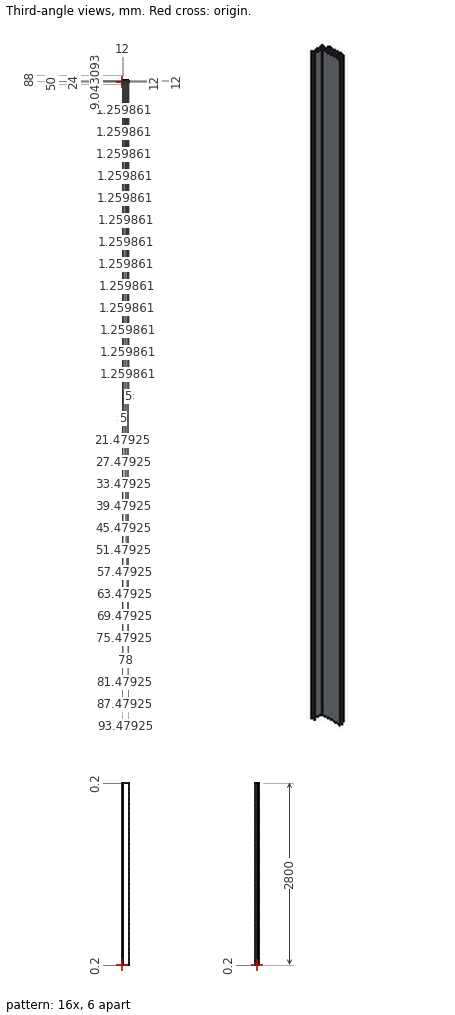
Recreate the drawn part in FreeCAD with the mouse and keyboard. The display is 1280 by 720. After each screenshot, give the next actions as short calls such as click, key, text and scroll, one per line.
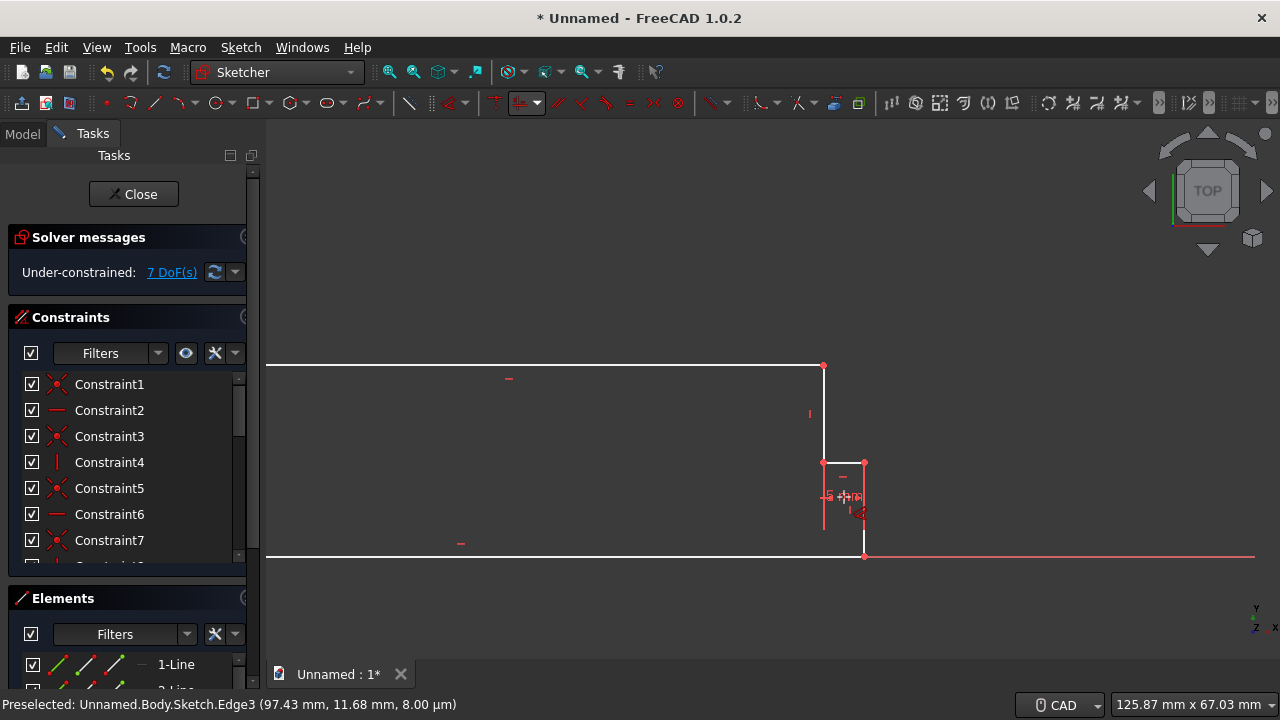
scroll(902, 581, down, 4)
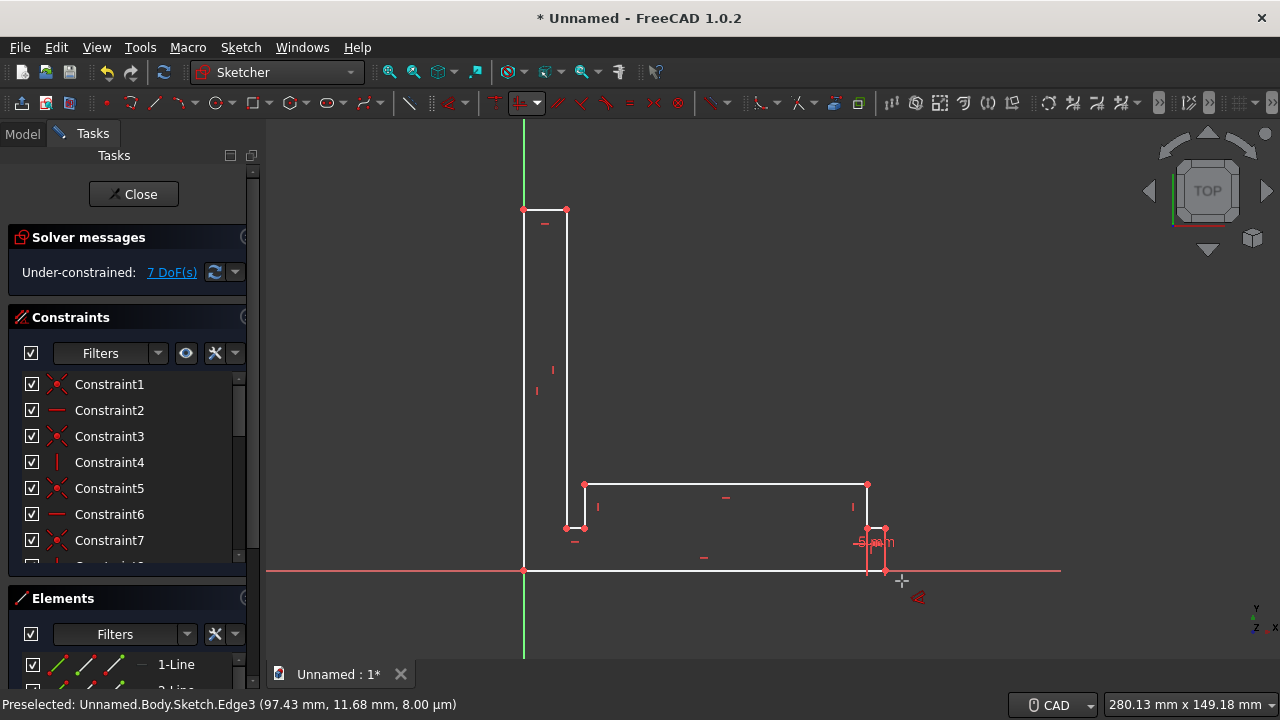
scroll(579, 528, up, 5)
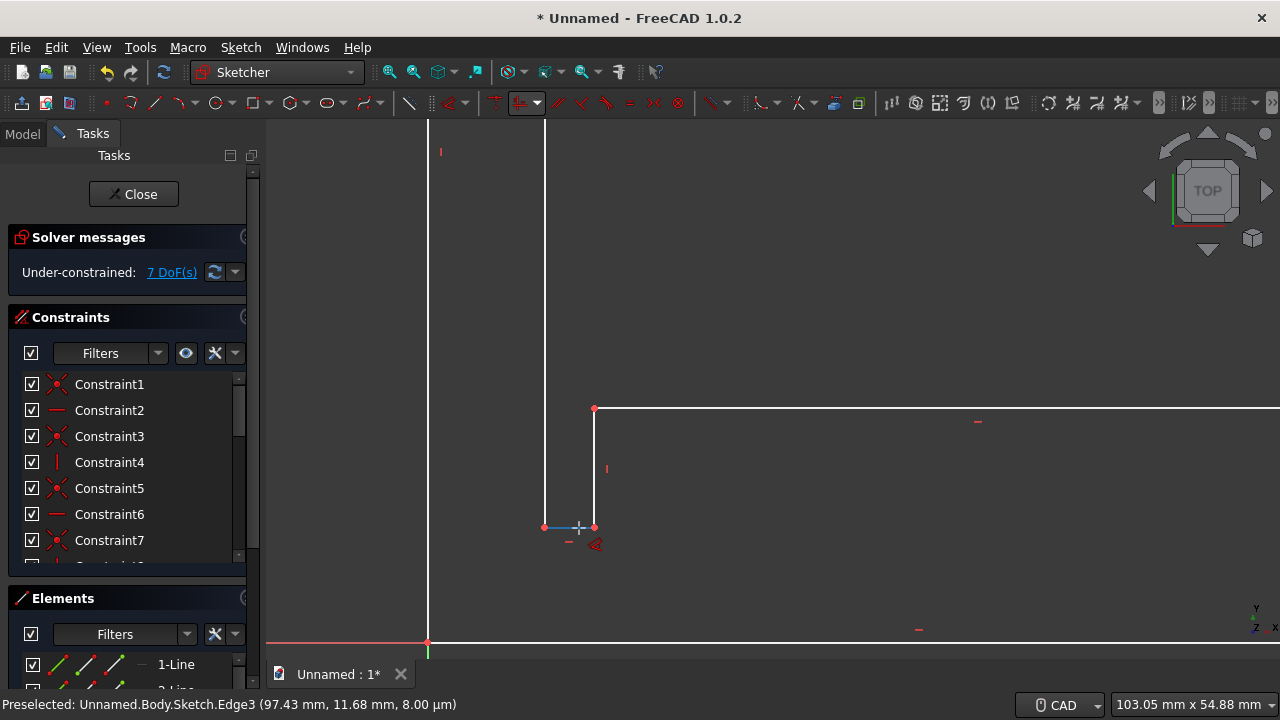
click(579, 528)
click(569, 562)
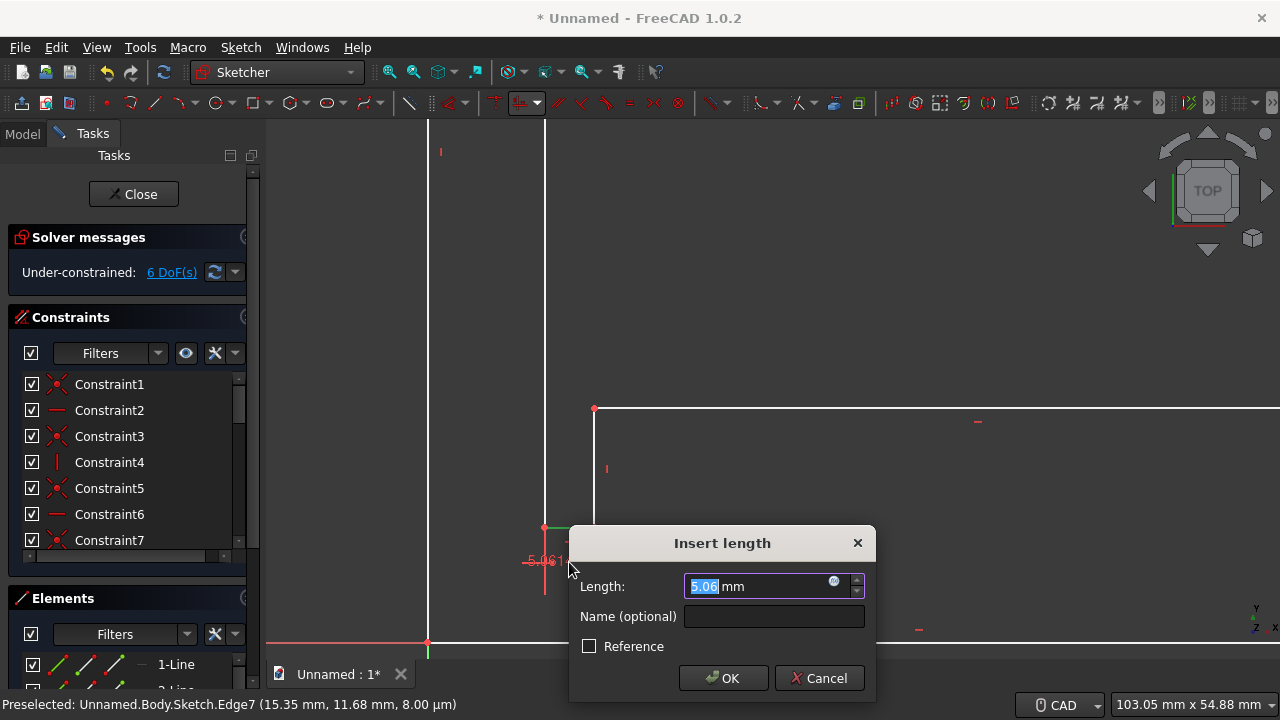
text(5)
key(Return)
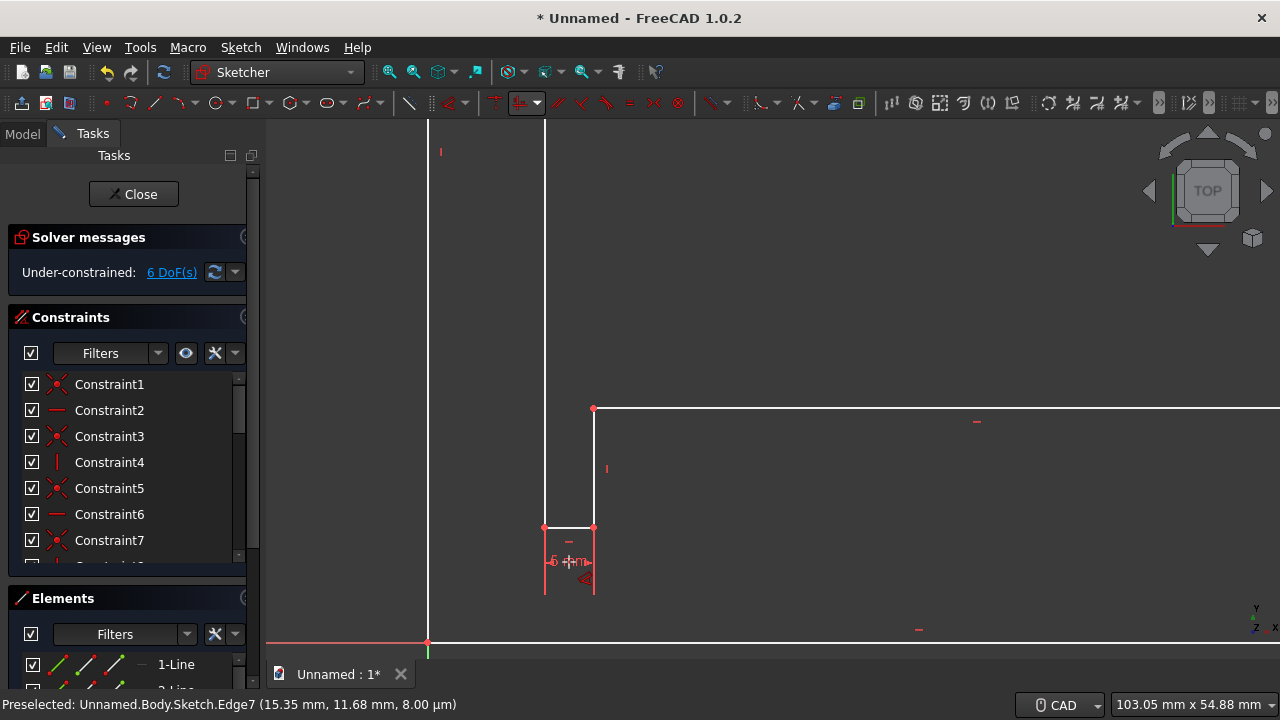
scroll(579, 528, down, 5)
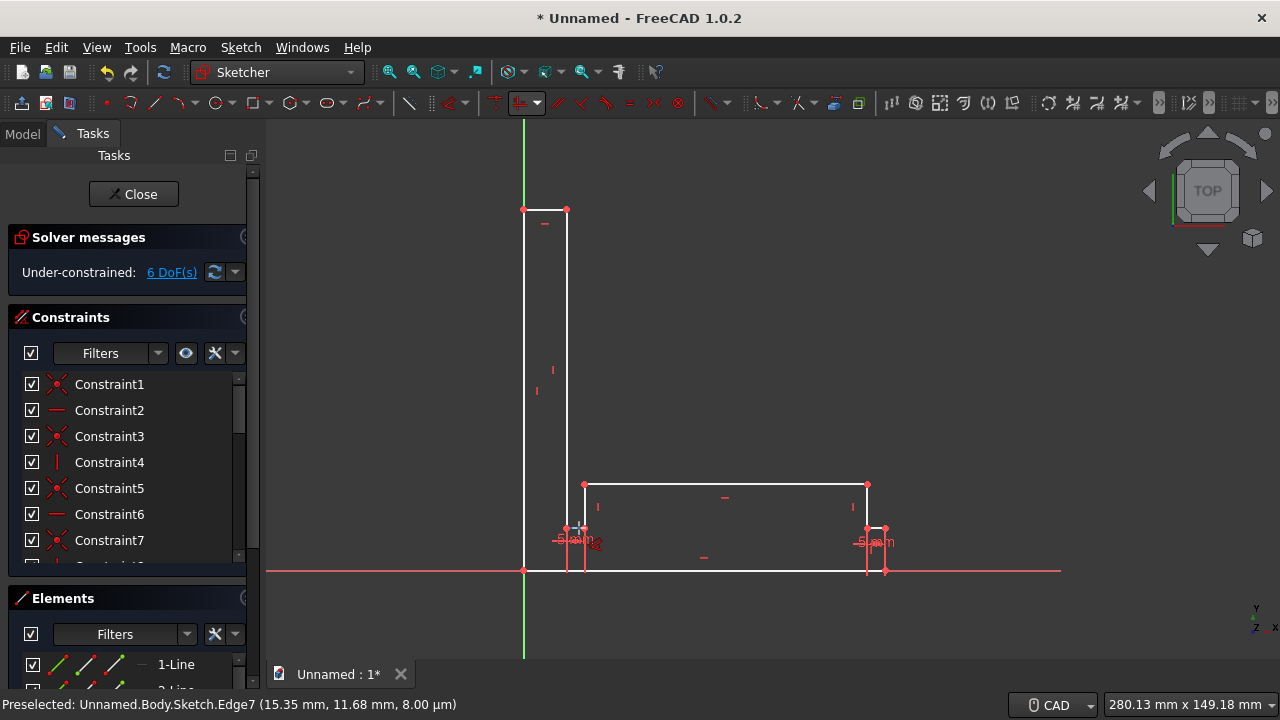
click(885, 558)
click(967, 550)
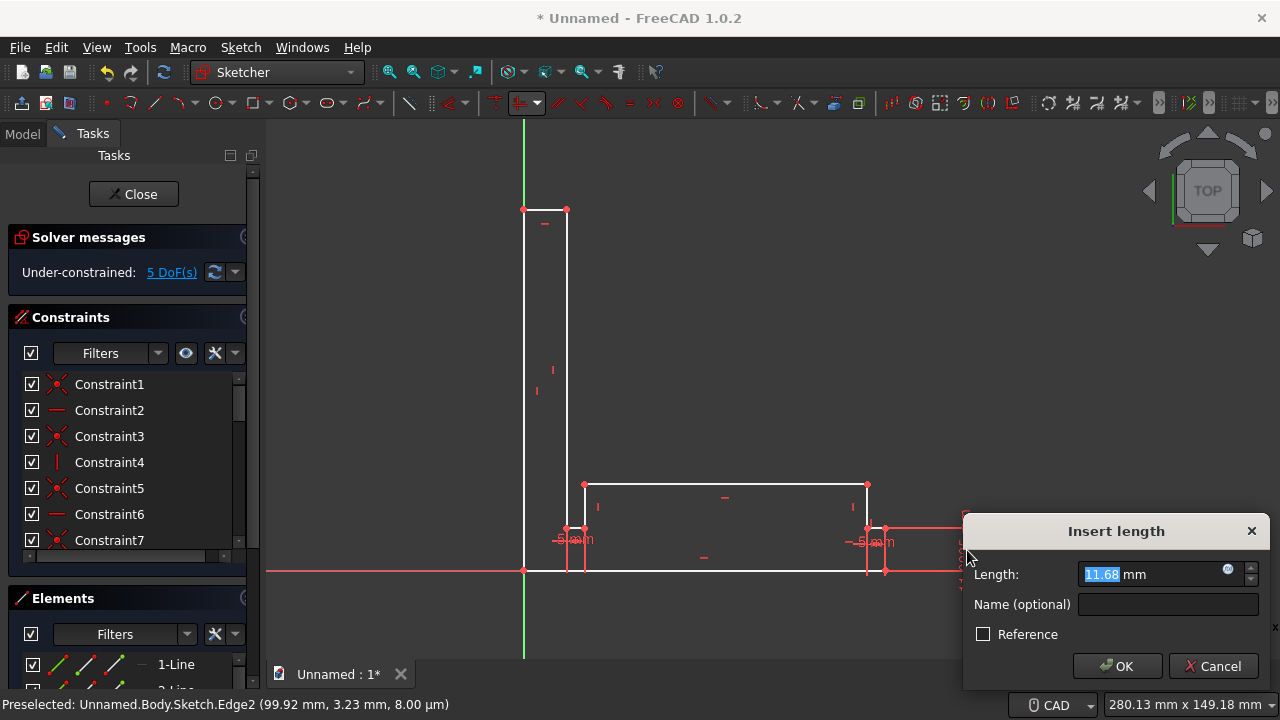
text(12)
key(Return)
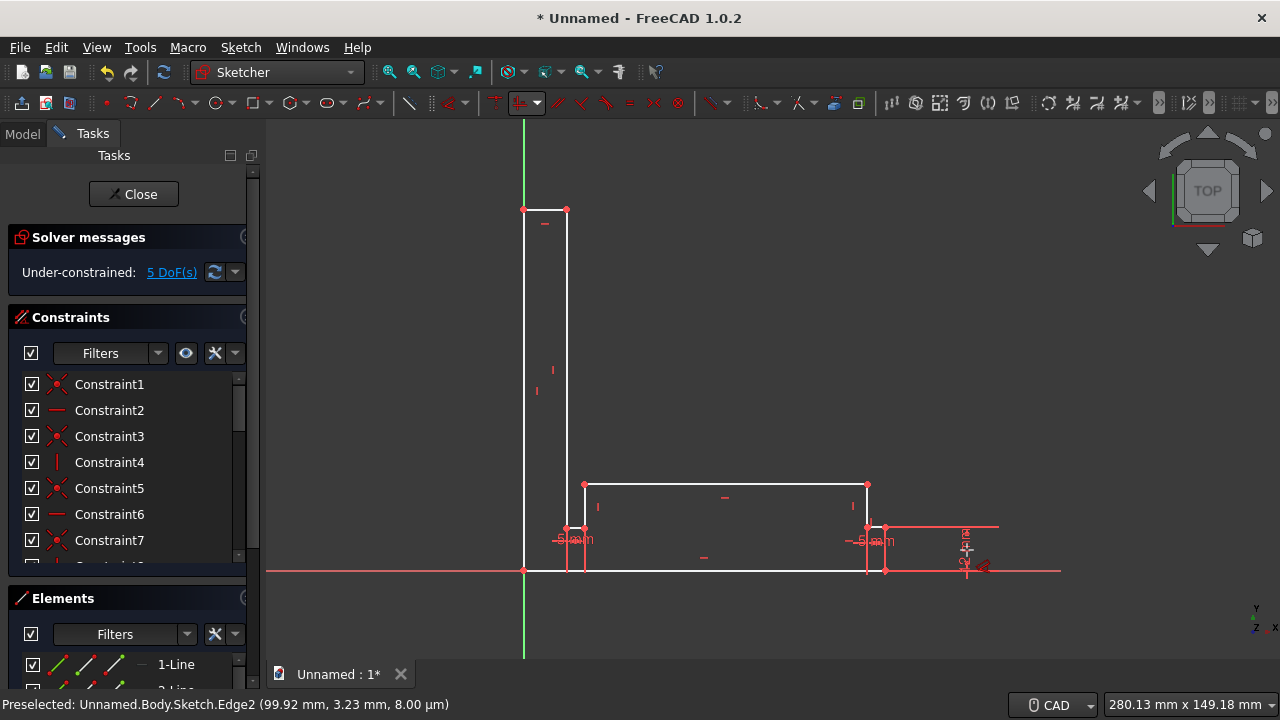
click(867, 514)
click(901, 506)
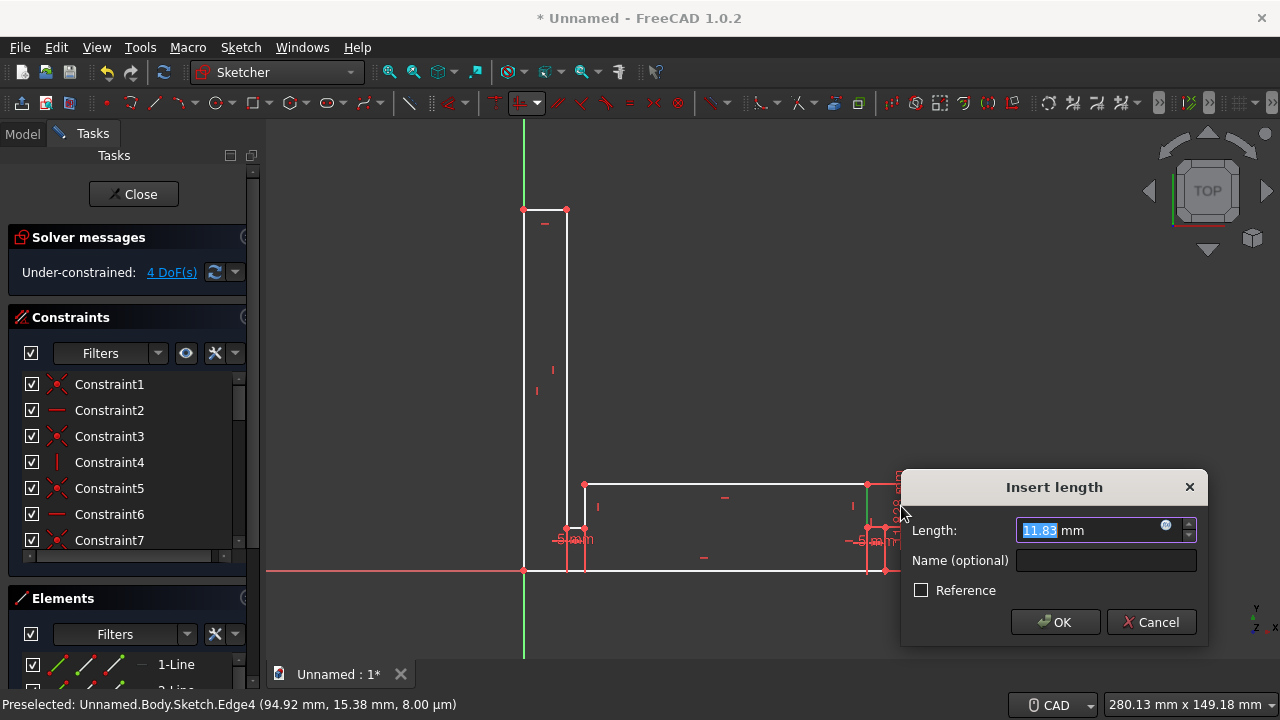
text(12)
key(Return)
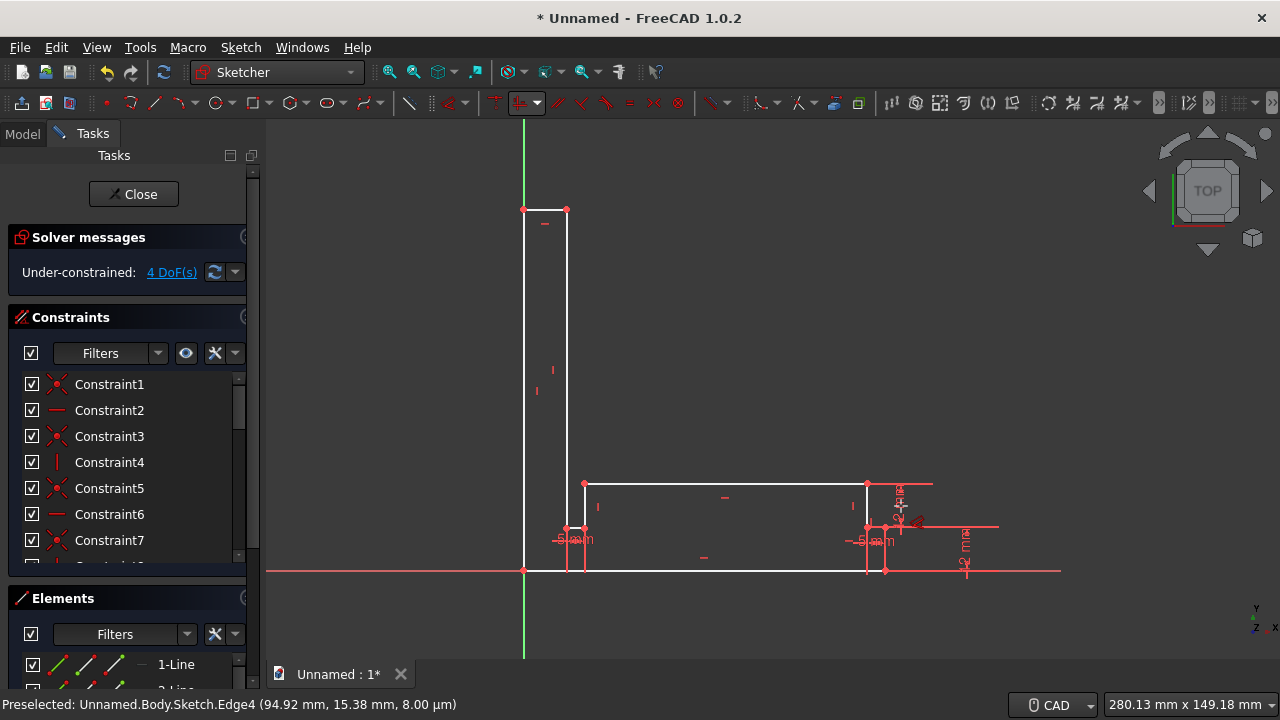
click(782, 484)
click(726, 518)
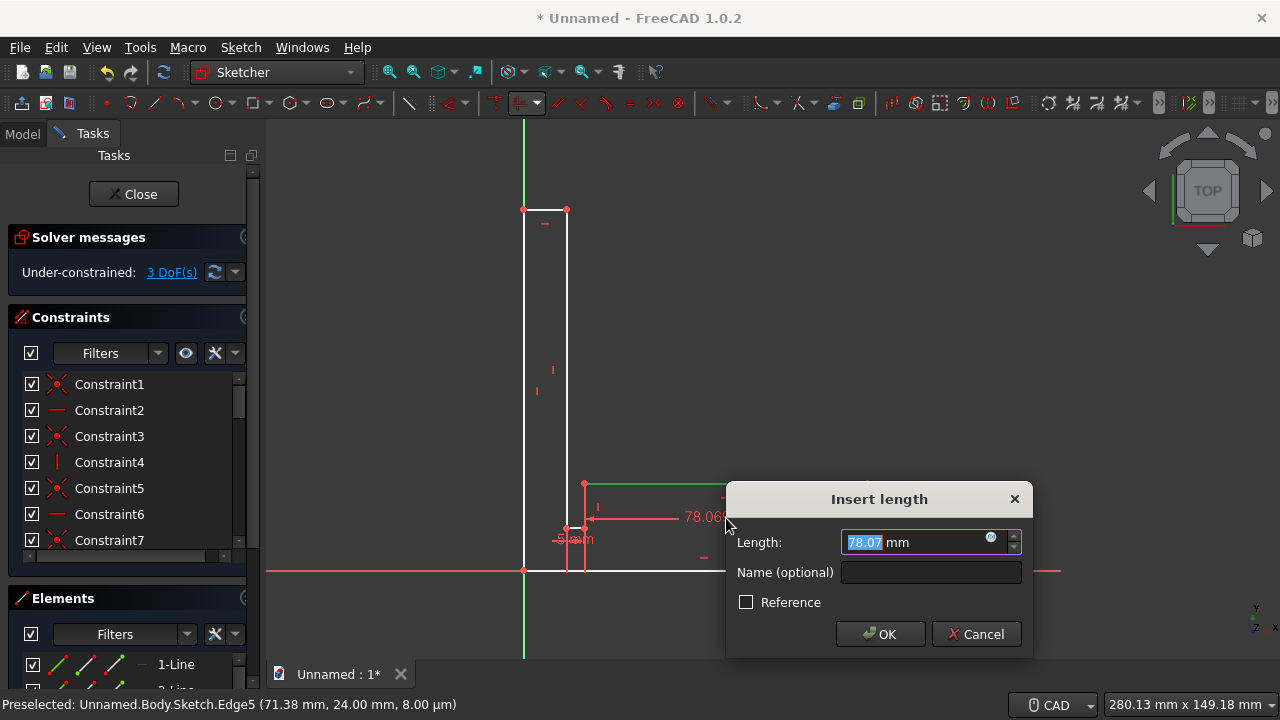
text(78)
key(Return)